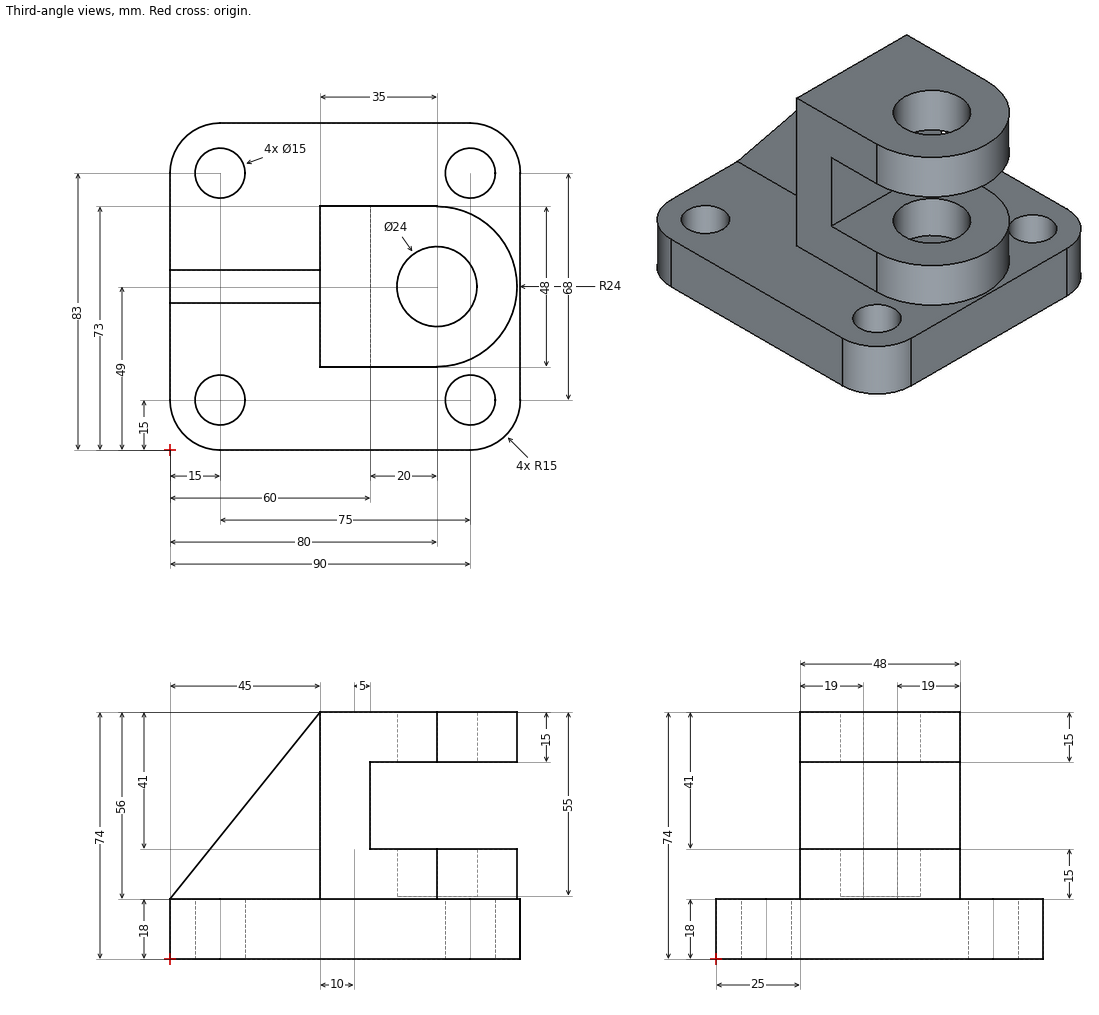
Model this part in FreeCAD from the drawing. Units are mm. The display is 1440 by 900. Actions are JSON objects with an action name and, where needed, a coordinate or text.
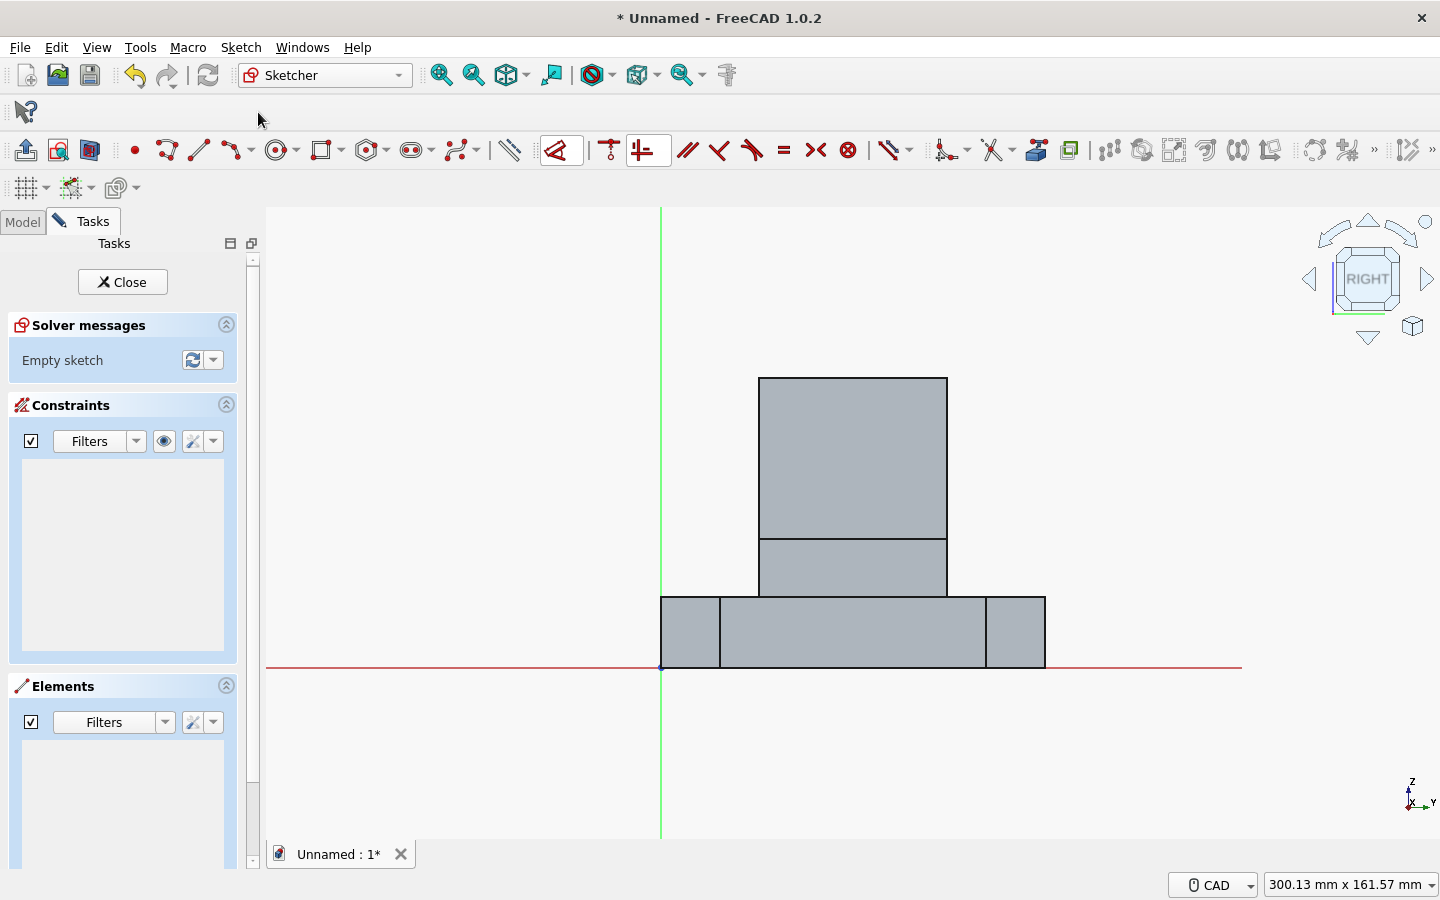
{"action": "left_click", "coordinate": [90, 150]}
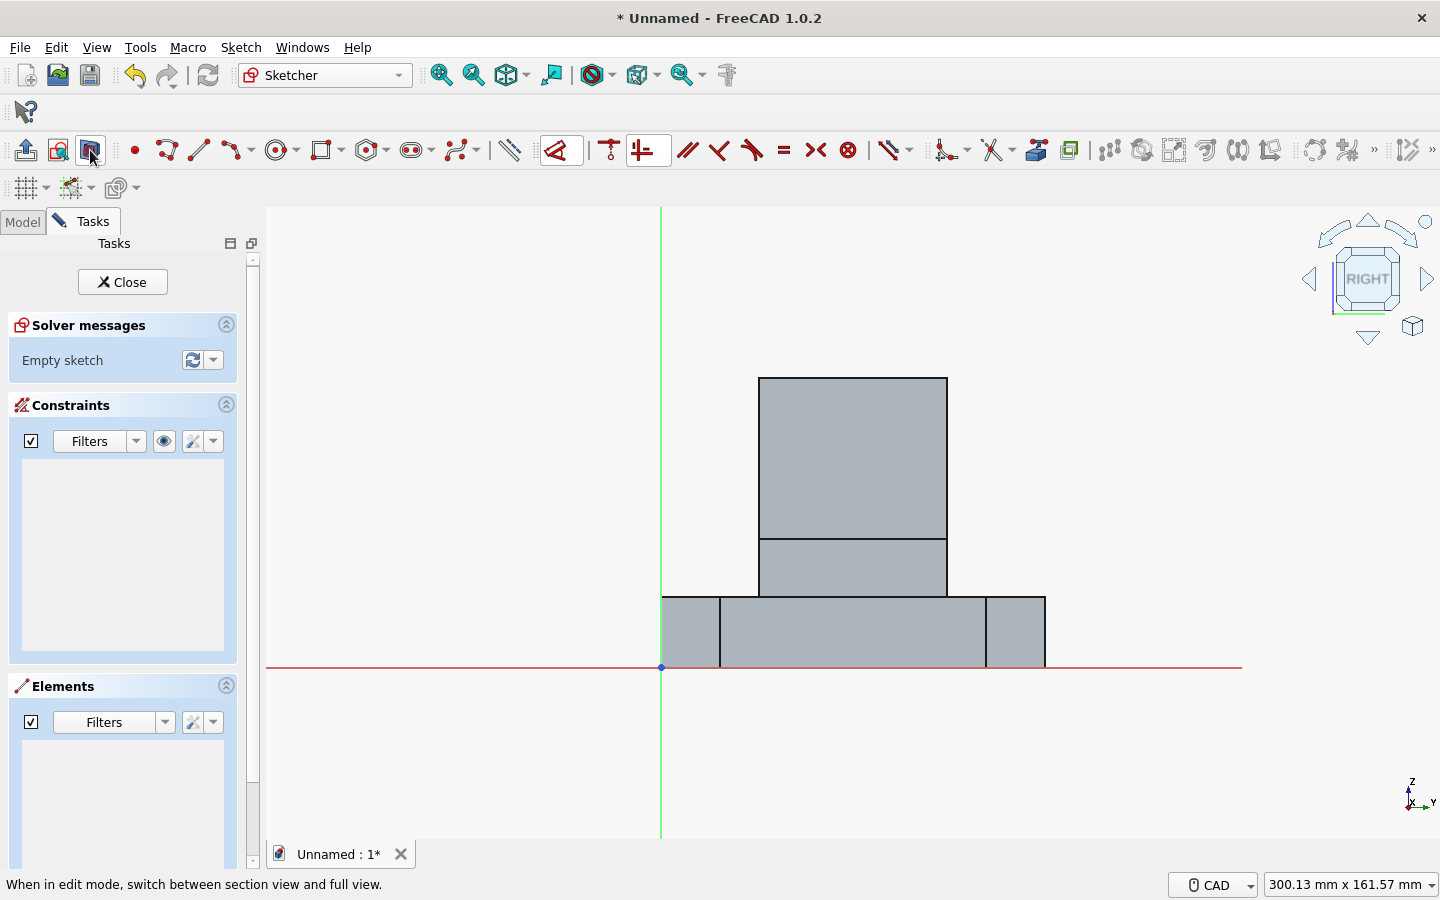
{"action": "scroll", "coordinate": [844, 523], "scroll_direction": "up", "scroll_amount": 2}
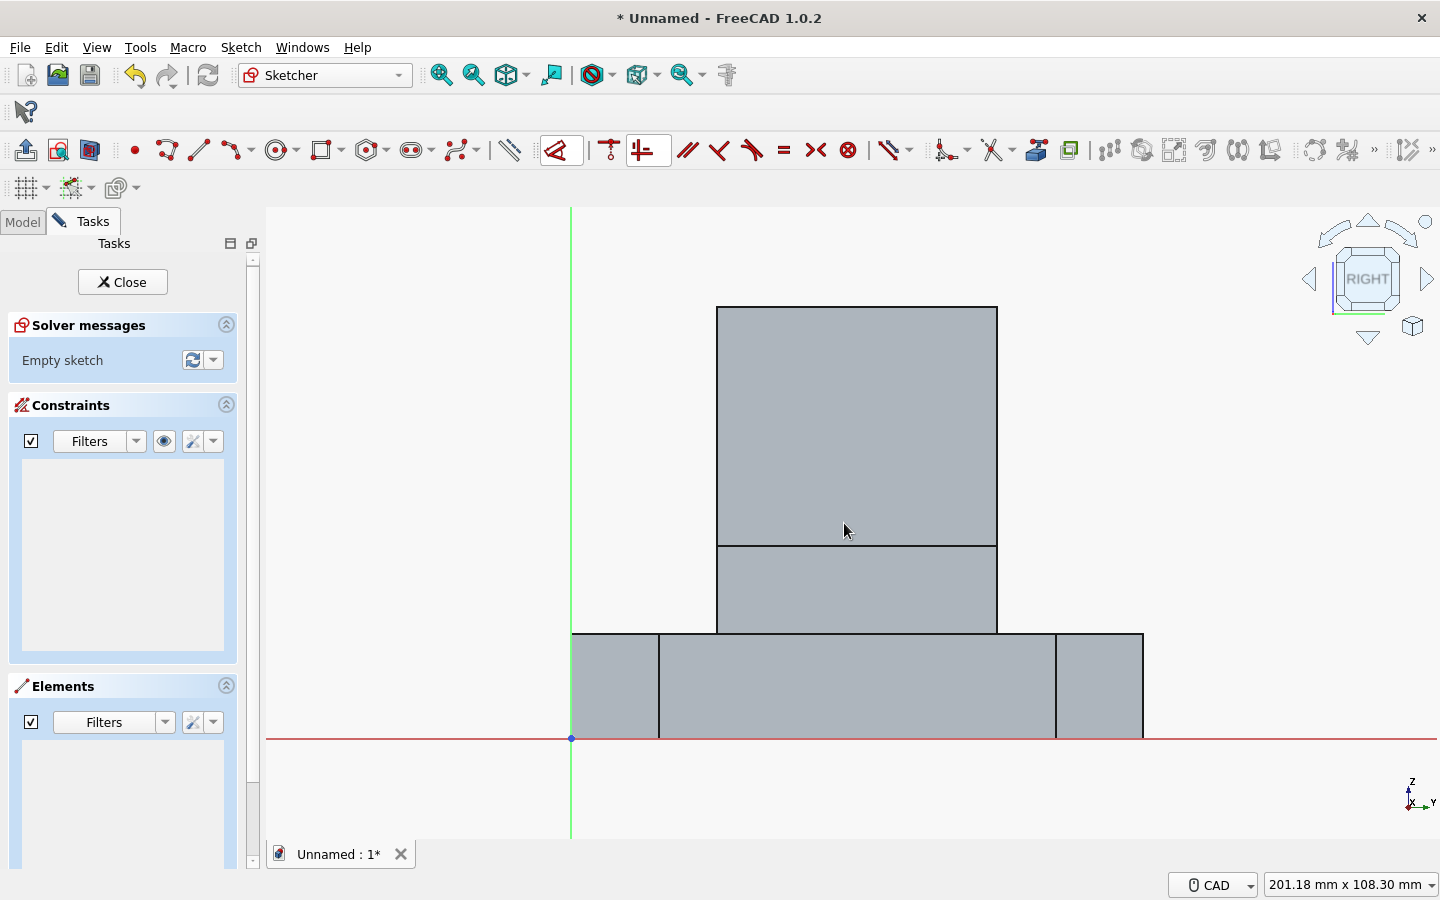
{"action": "left_click", "coordinate": [322, 150]}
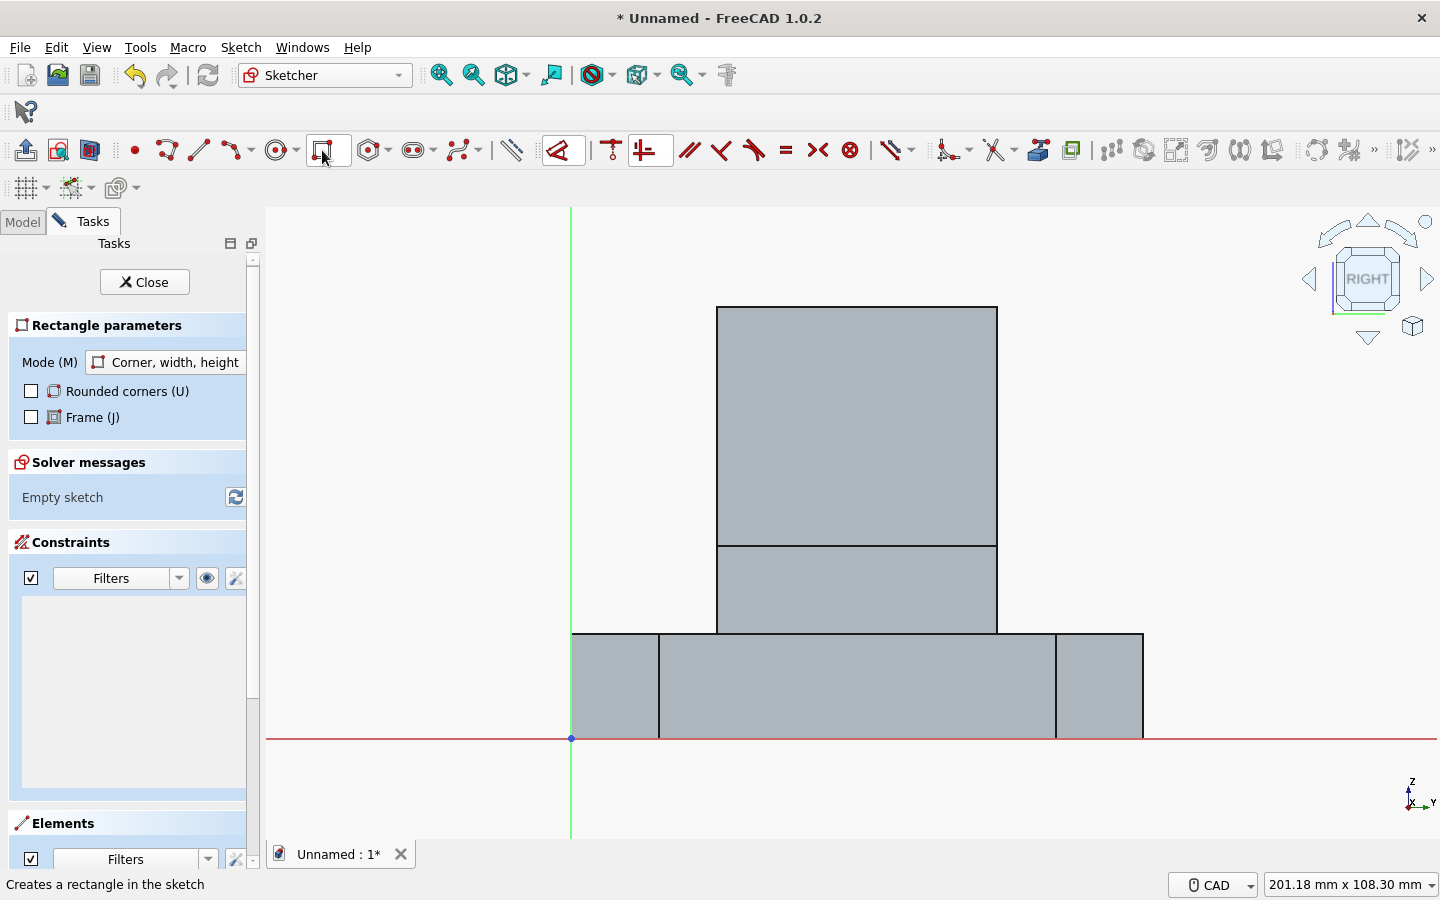
{"action": "left_click", "coordinate": [717, 307]}
{"action": "left_click", "coordinate": [997, 546]}
{"action": "key", "text": "Escape"}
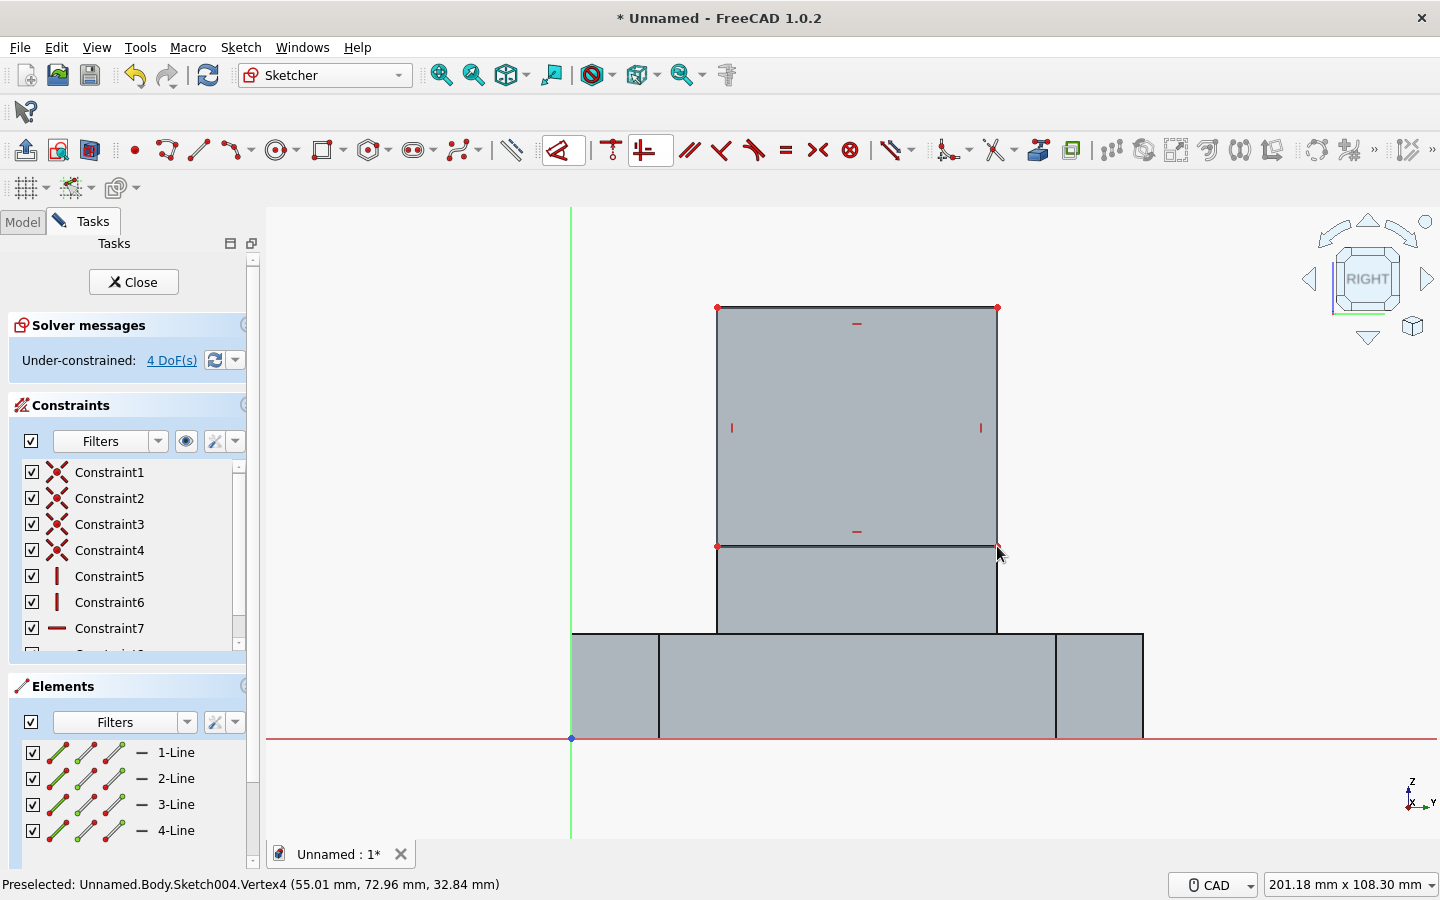
{"action": "left_click", "coordinate": [717, 380]}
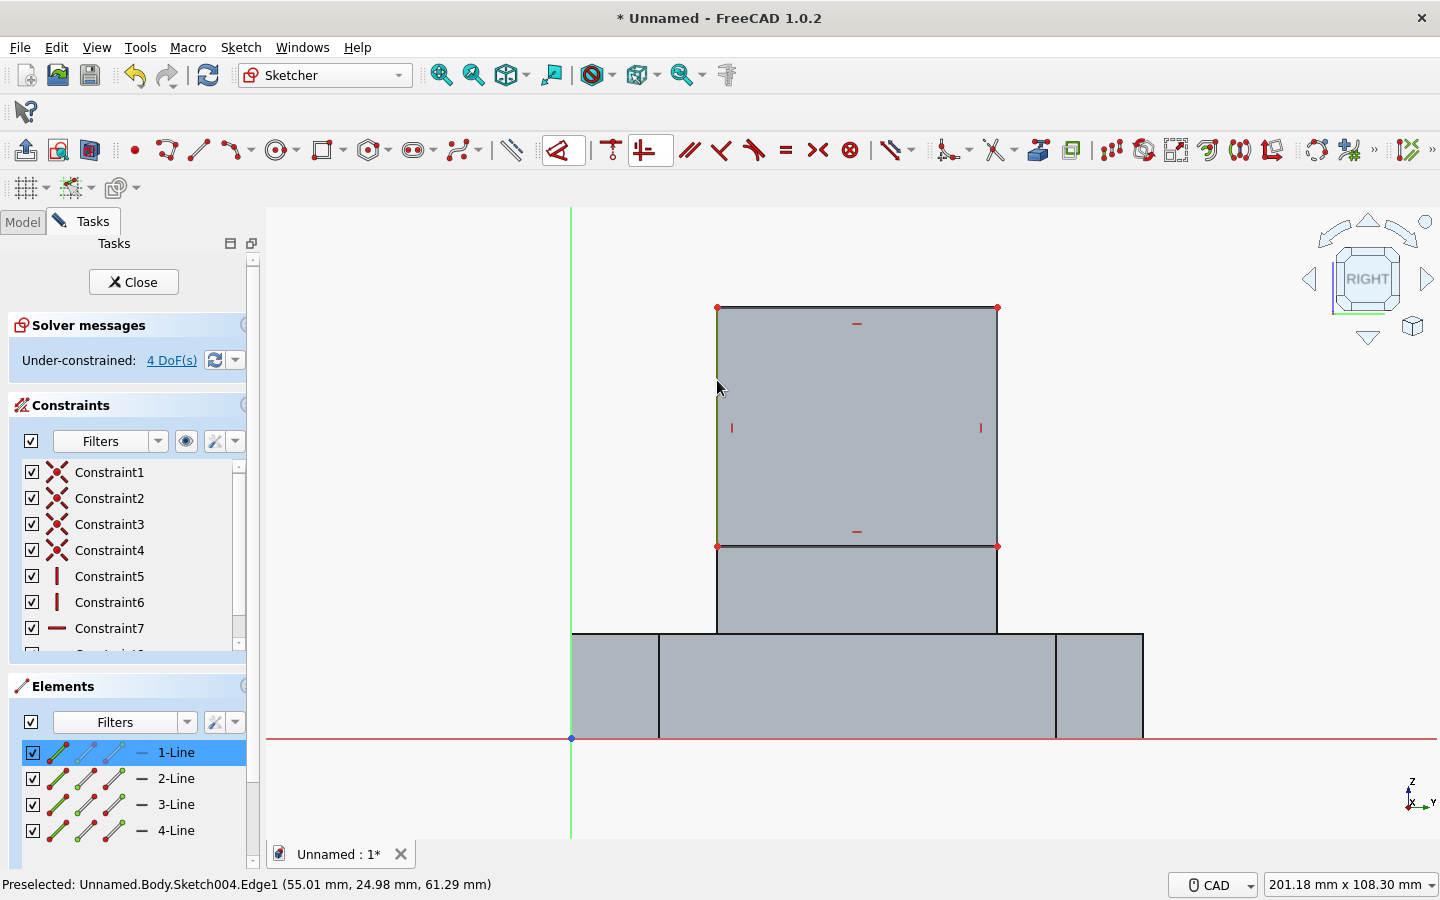
{"action": "left_click", "coordinate": [580, 150]}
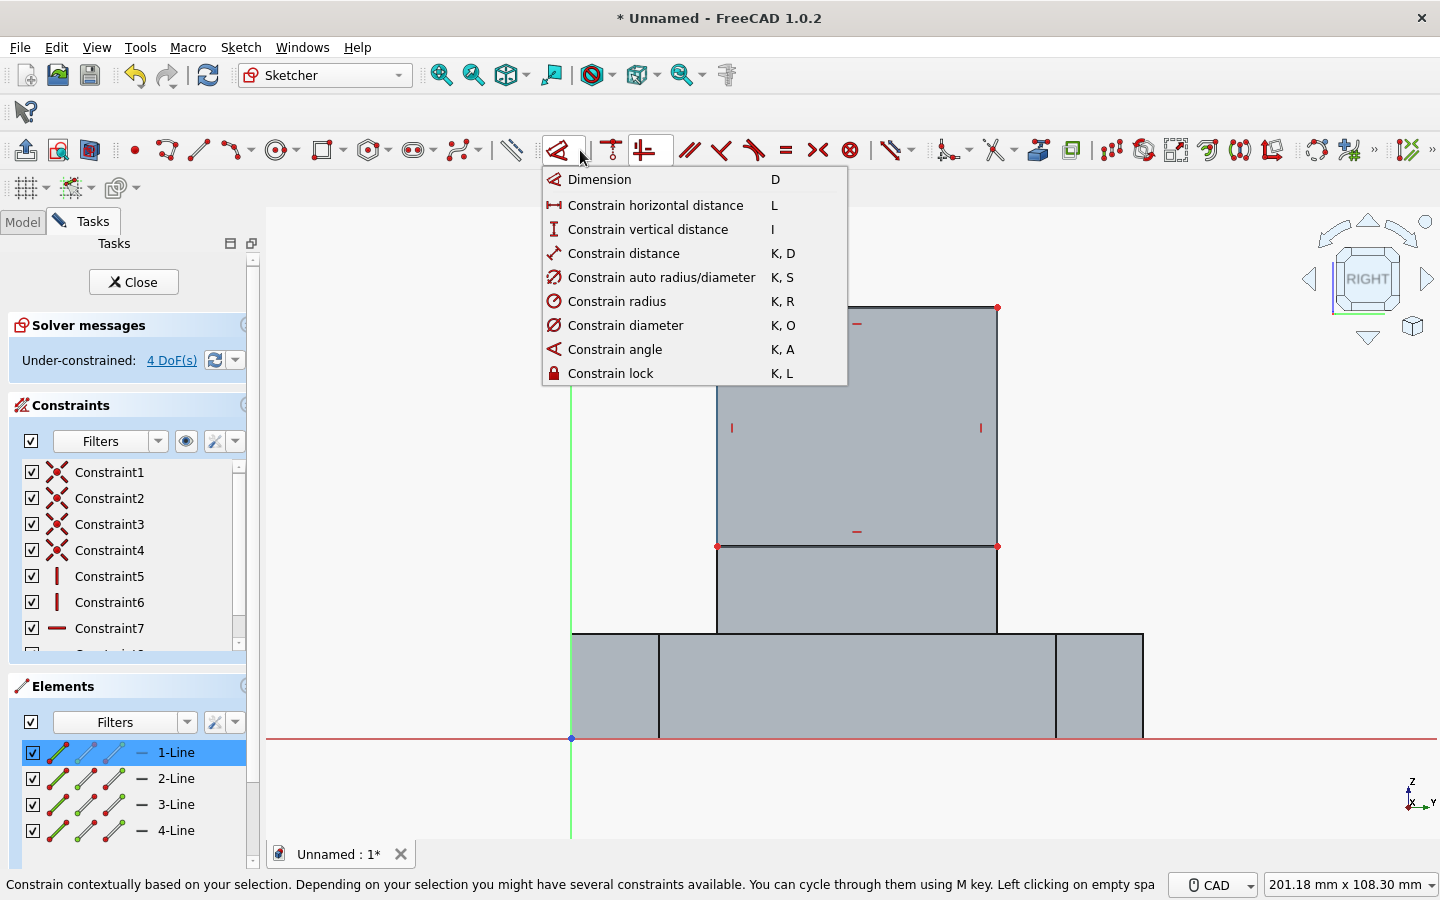
{"action": "left_click", "coordinate": [695, 229]}